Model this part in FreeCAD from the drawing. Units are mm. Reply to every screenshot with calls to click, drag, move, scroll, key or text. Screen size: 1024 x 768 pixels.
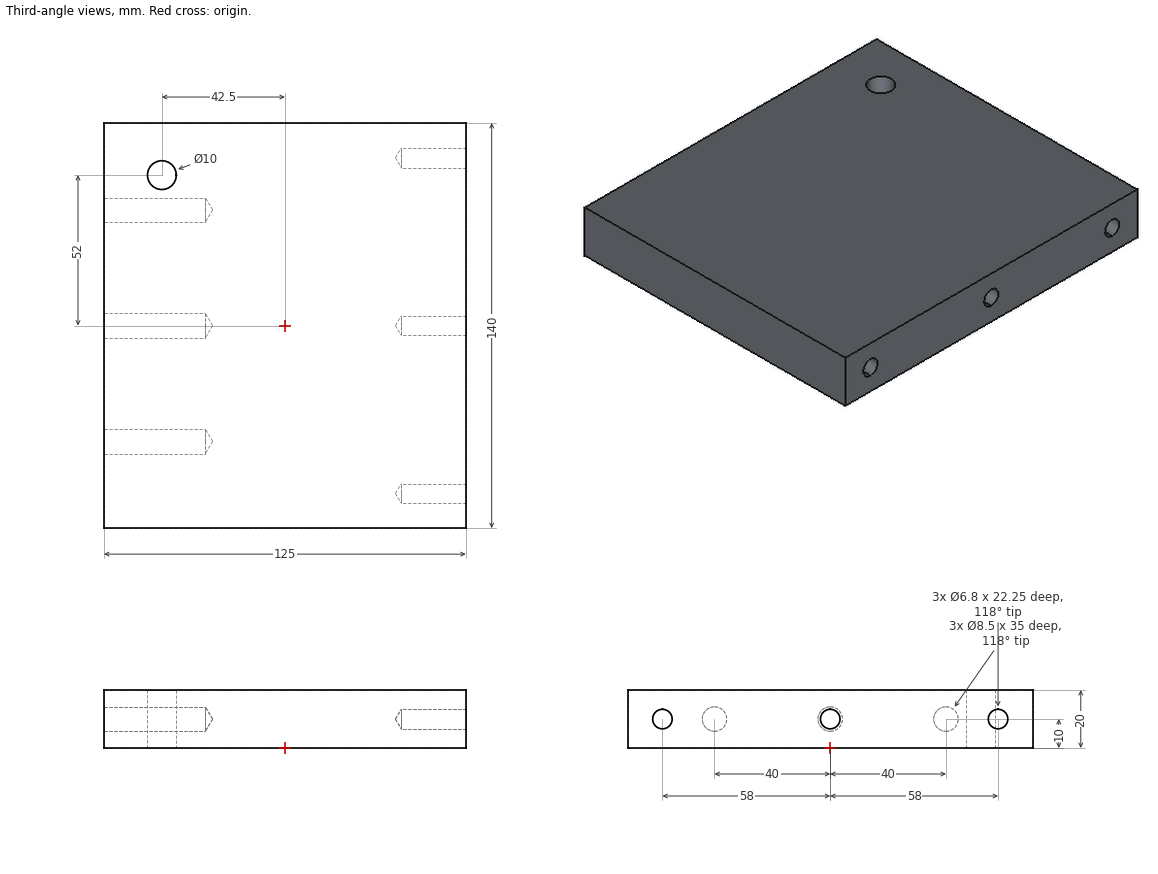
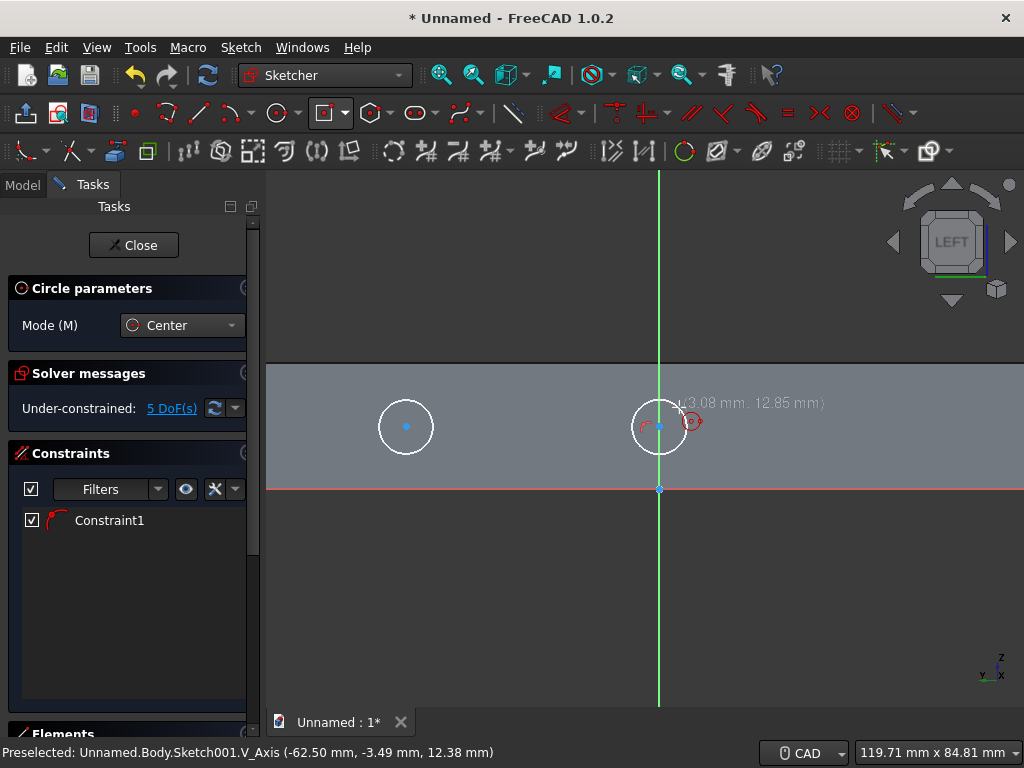
scroll(408, 427, down, 2)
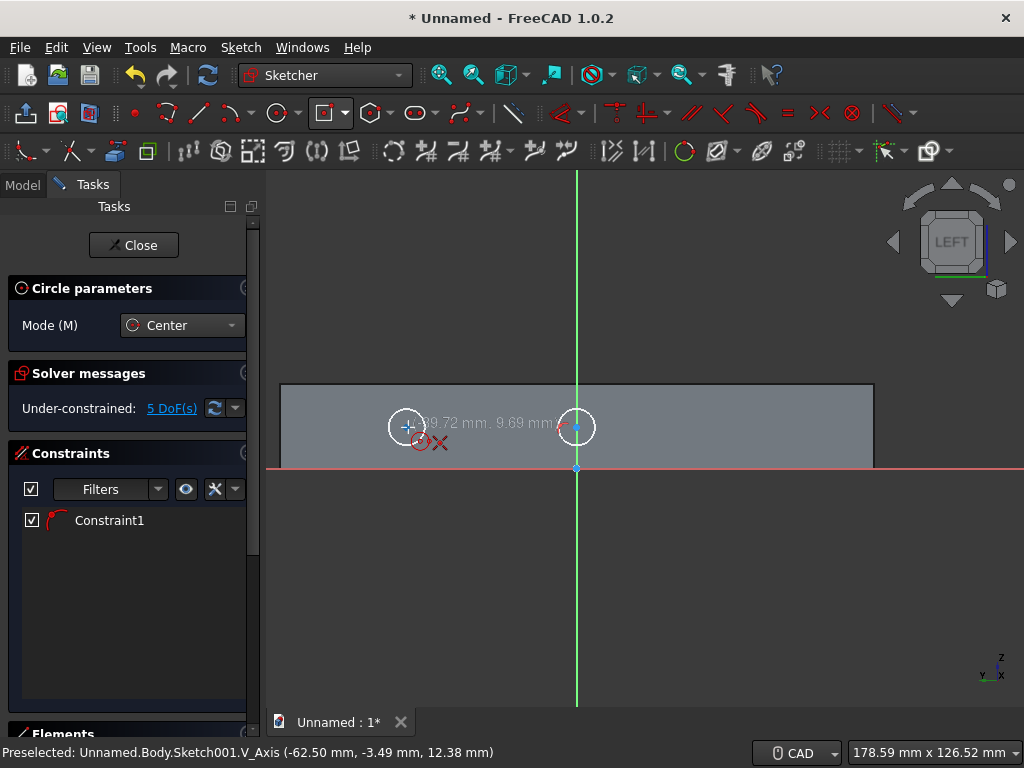
scroll(746, 427, up, 2)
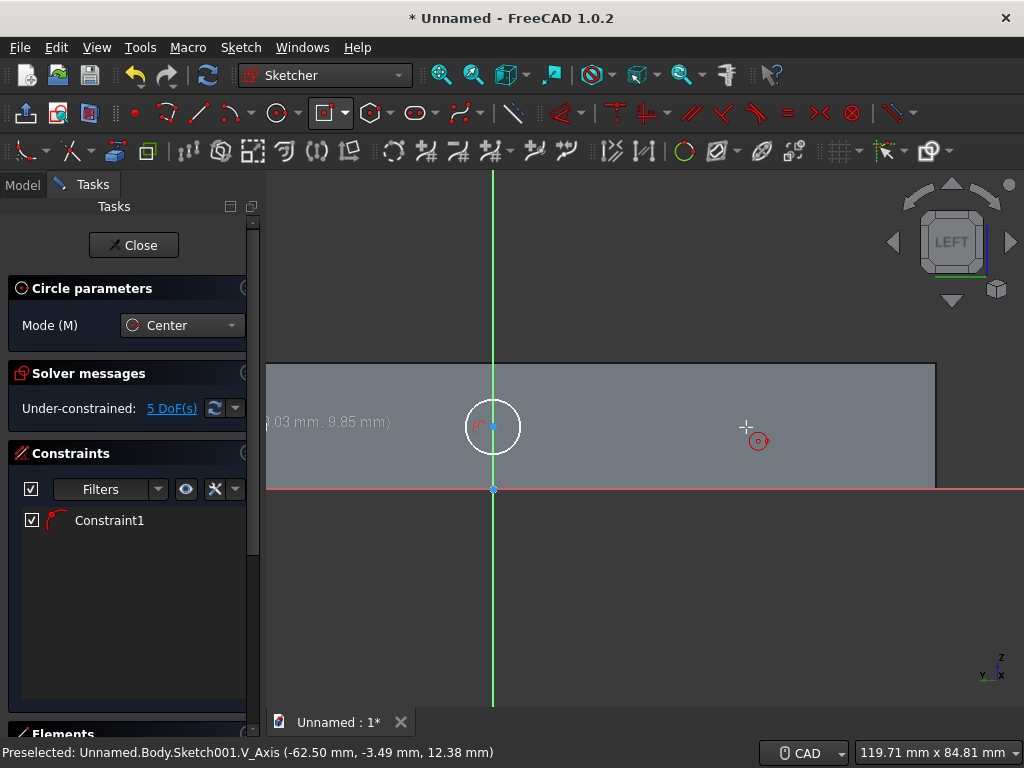
click(746, 426)
click(765, 407)
key(Escape)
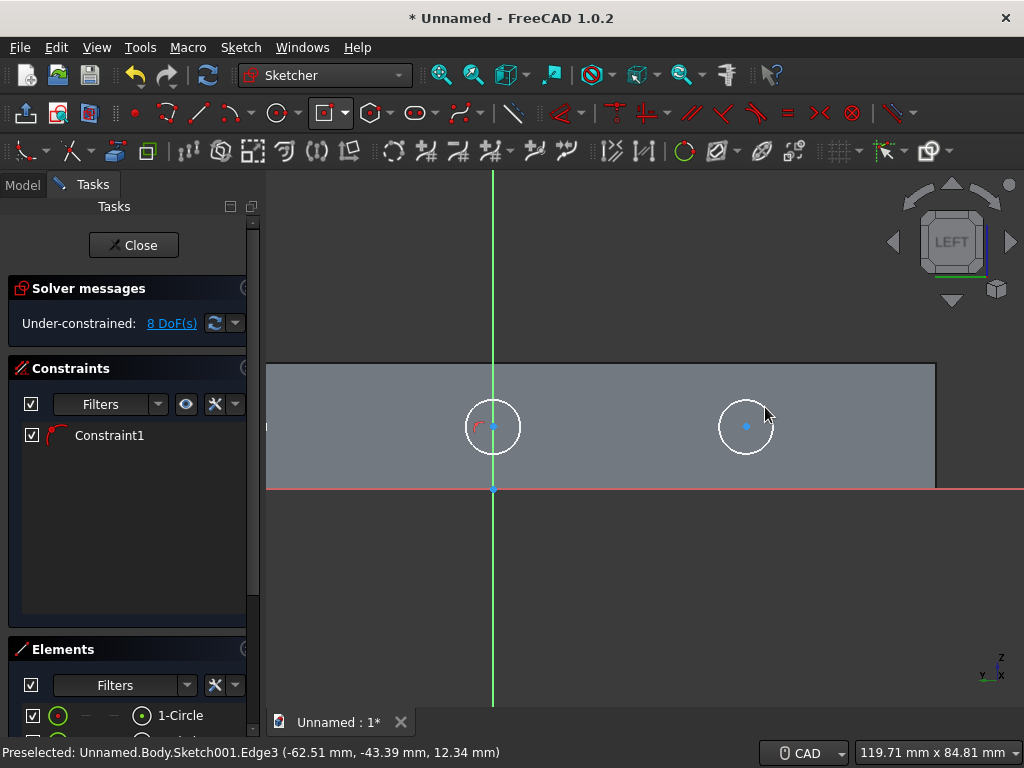
scroll(746, 427, down, 2)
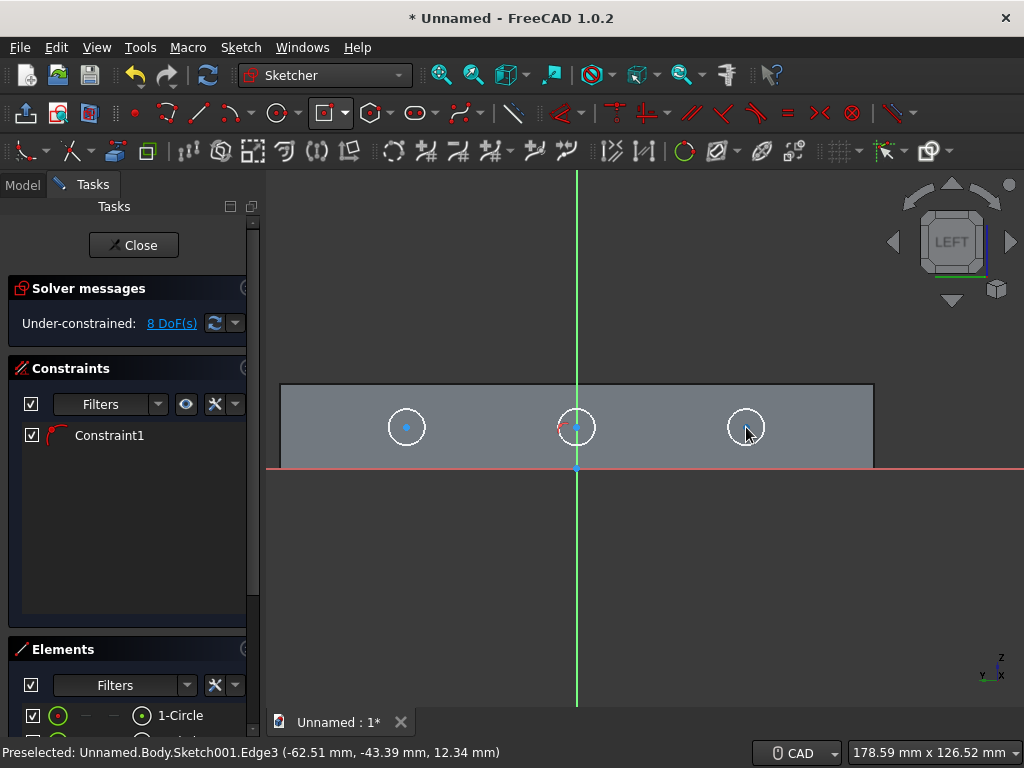
click(419, 414)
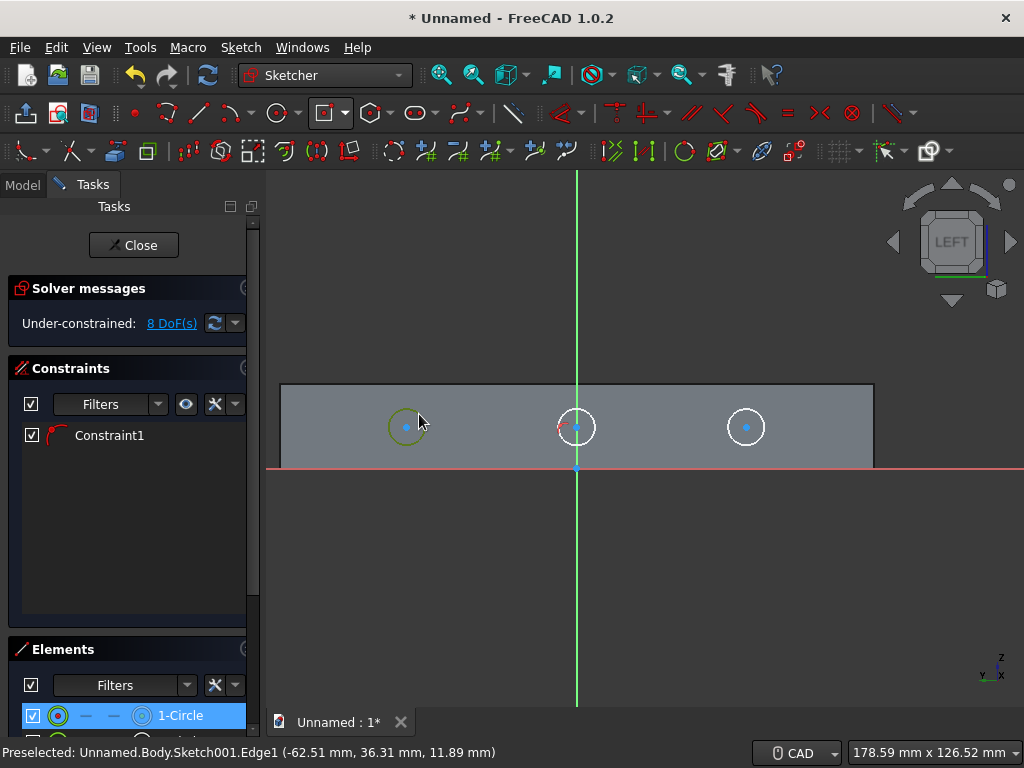
click(590, 414)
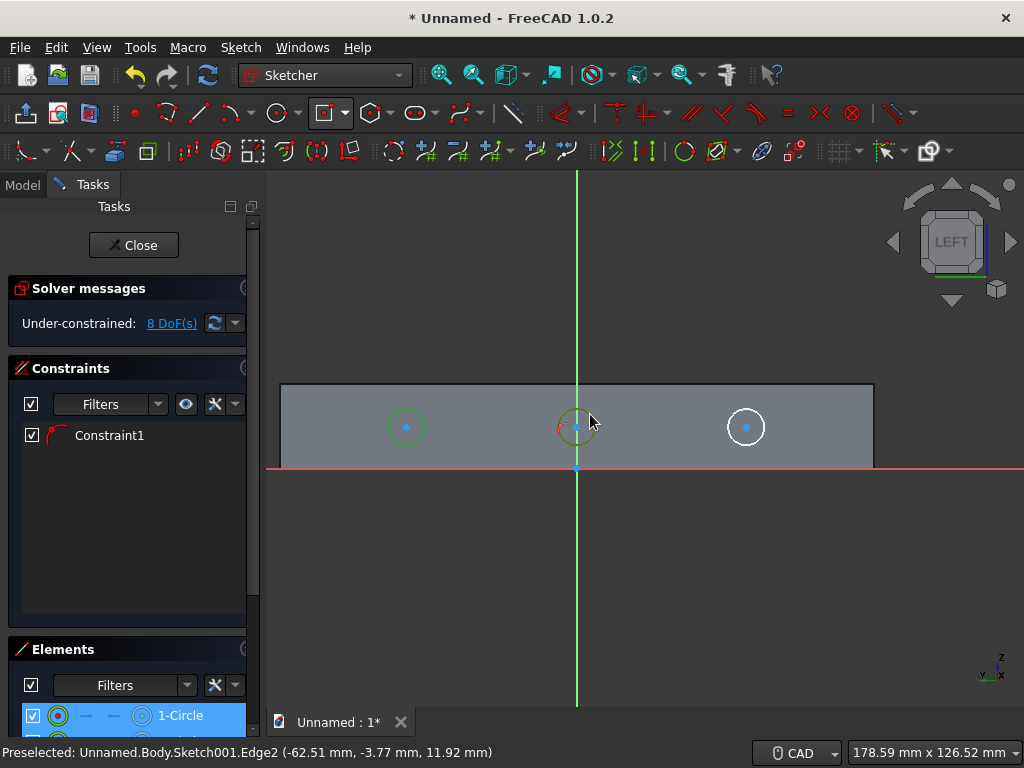
click(759, 414)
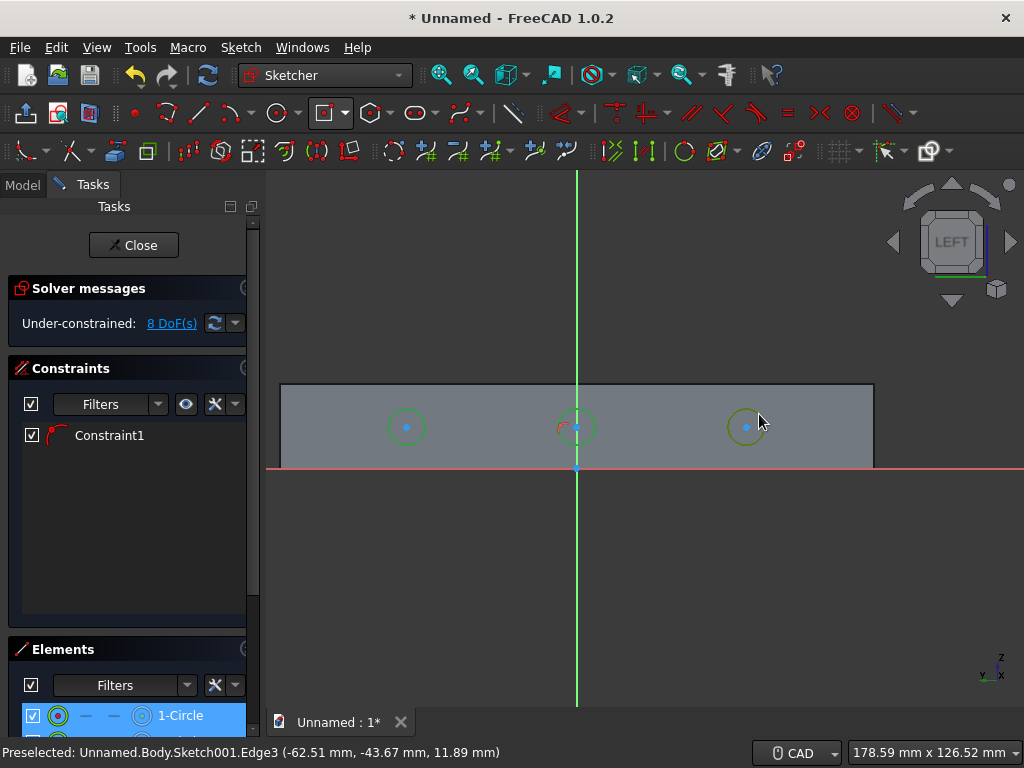
click(788, 114)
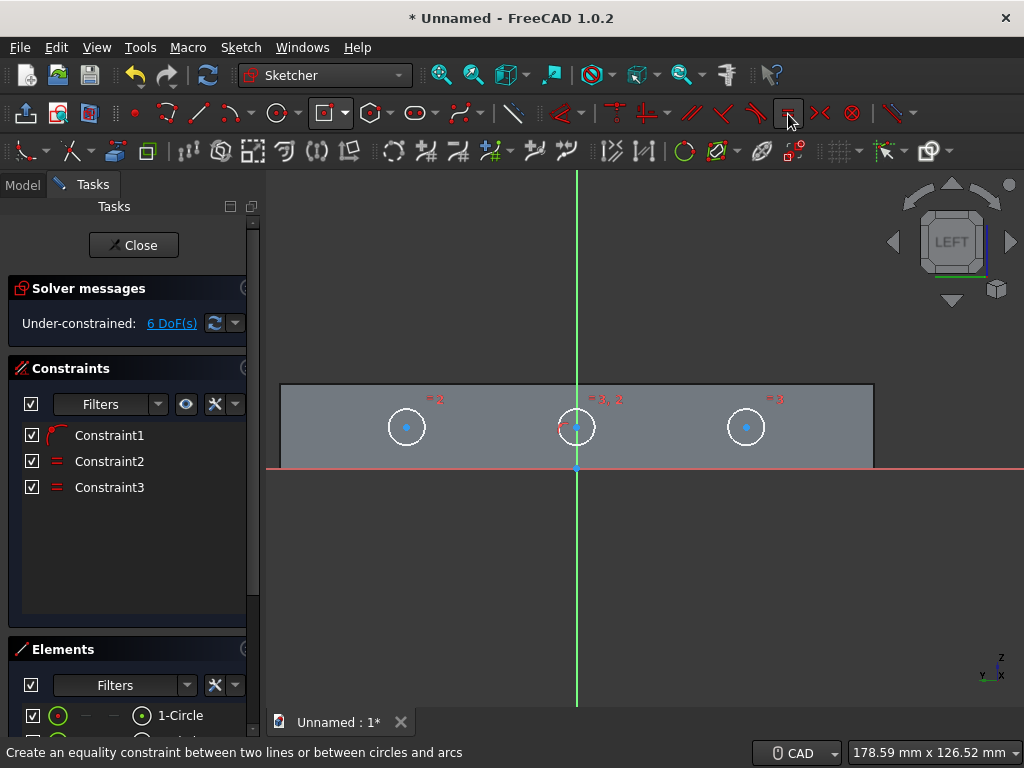
click(407, 427)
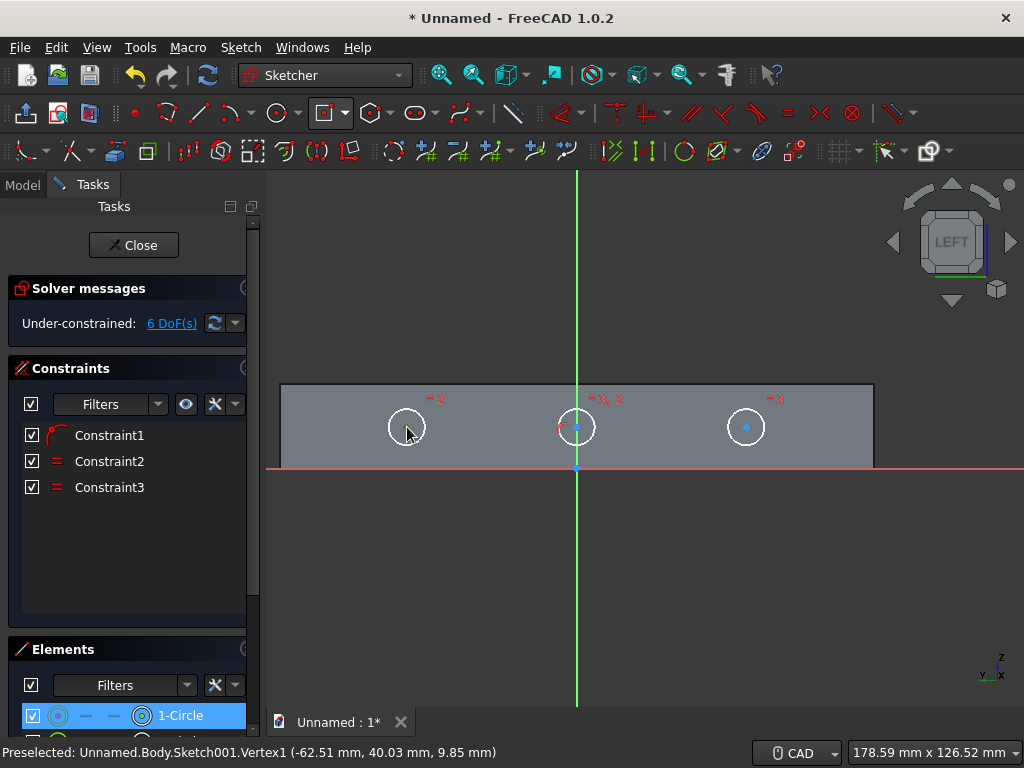
click(577, 427)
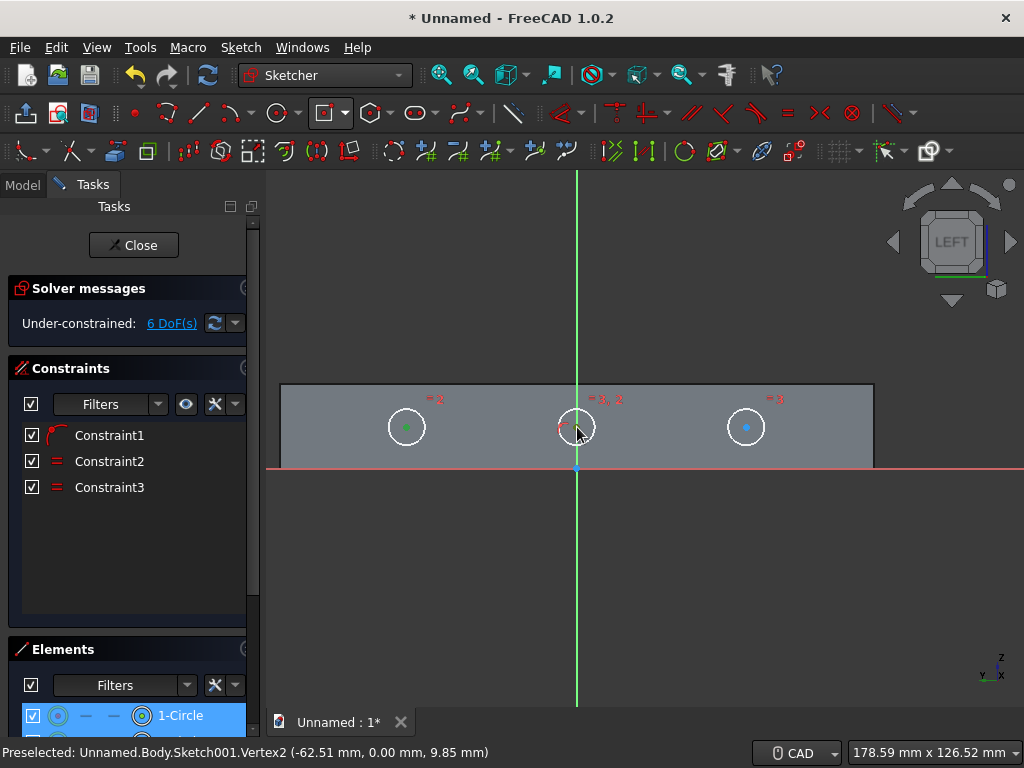
click(670, 114)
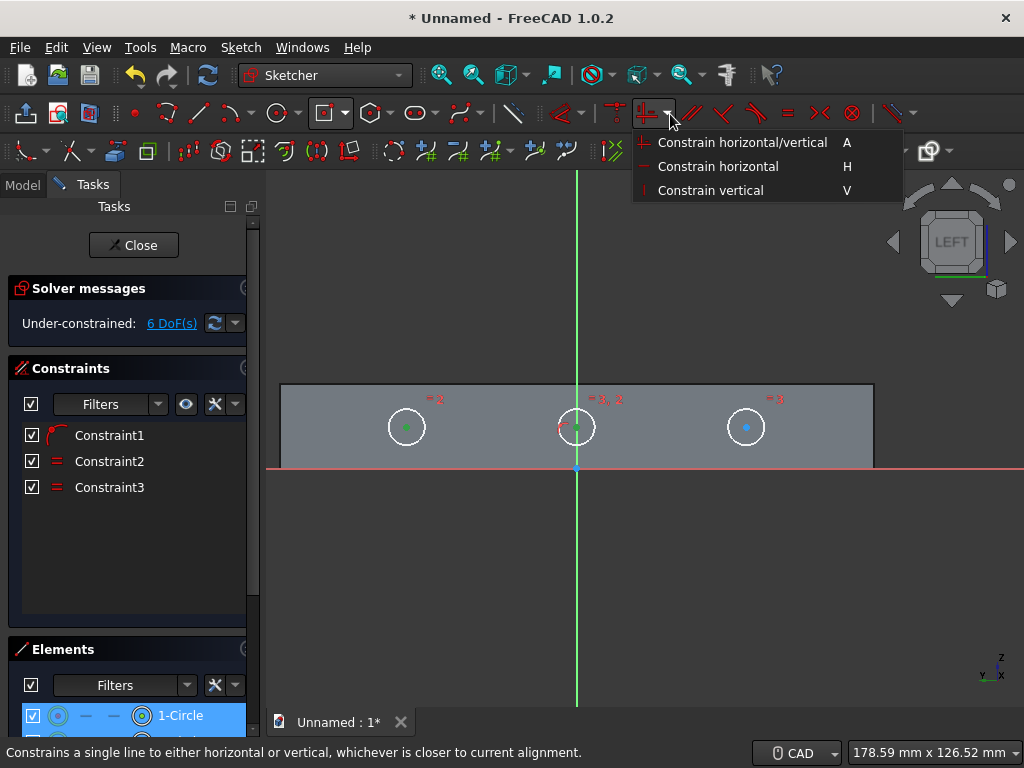
click(768, 166)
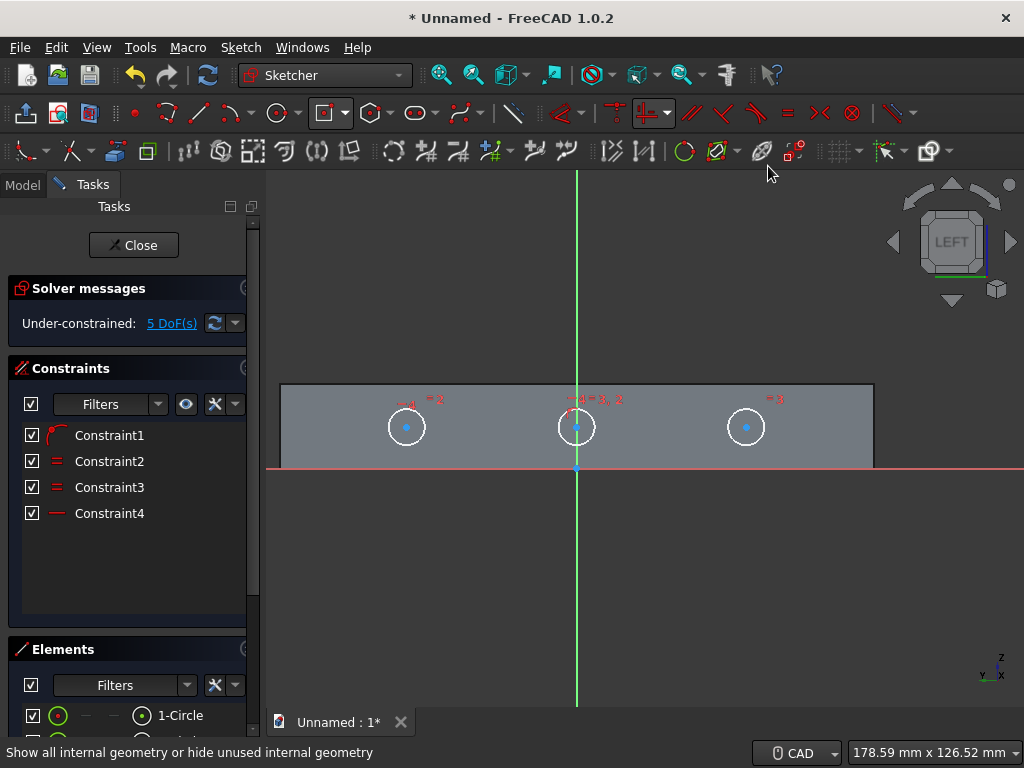
click(577, 427)